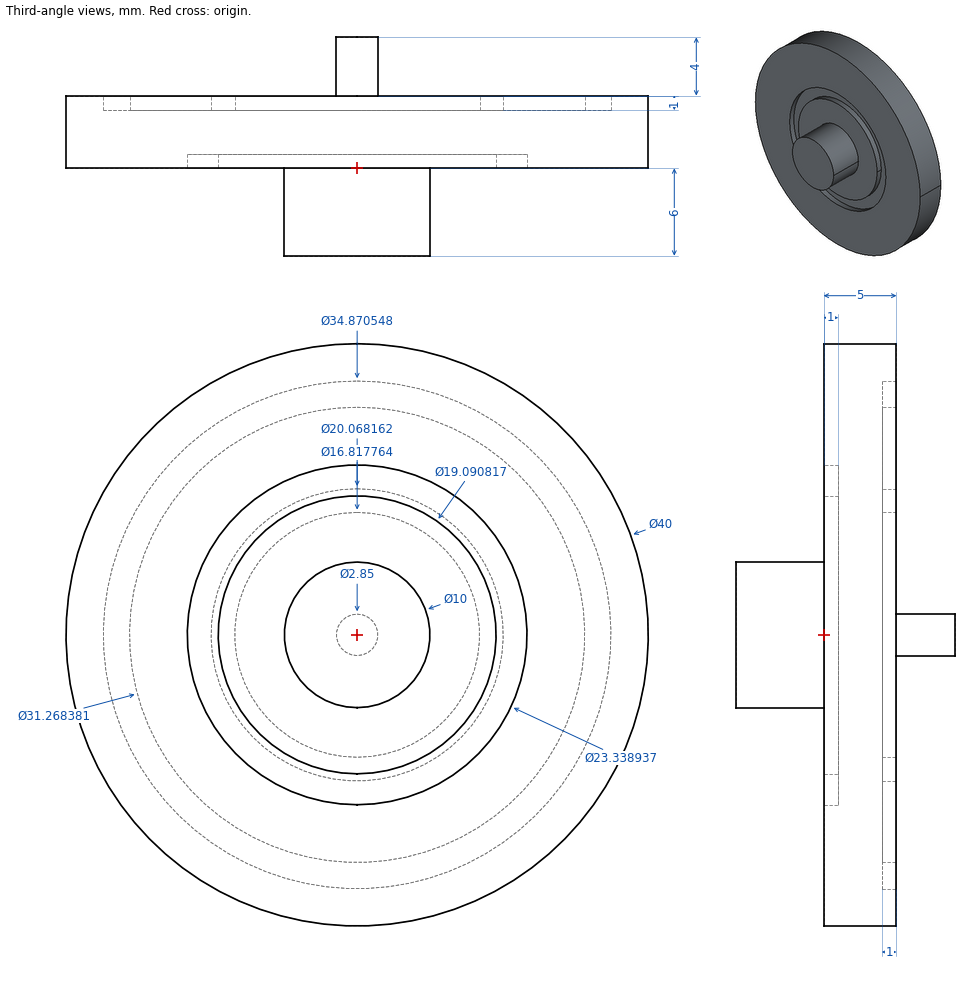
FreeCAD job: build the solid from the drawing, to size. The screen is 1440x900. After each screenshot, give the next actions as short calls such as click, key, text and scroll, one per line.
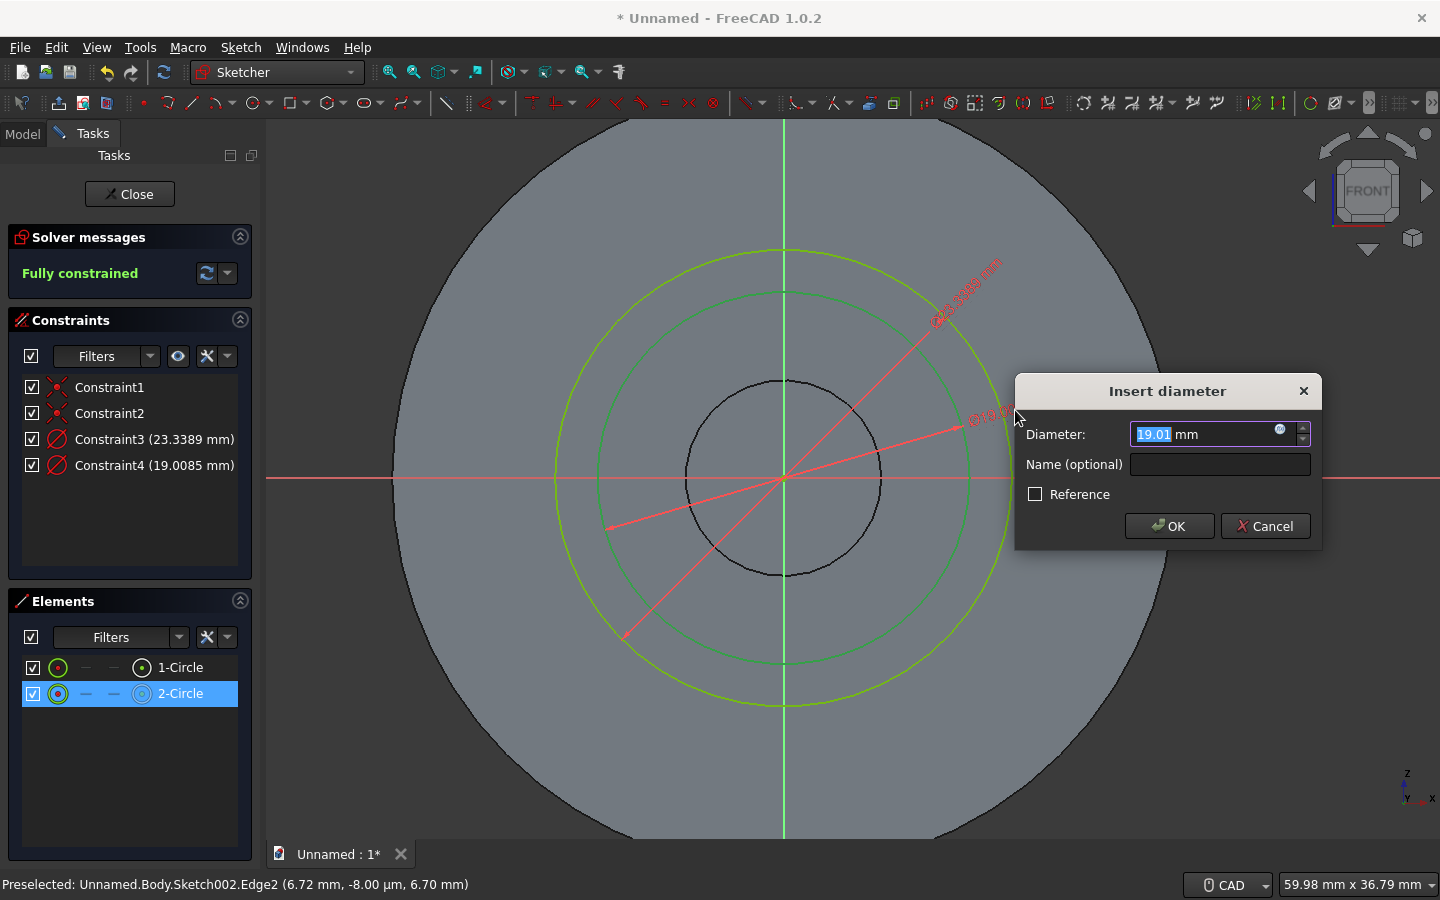
text(19.090817)
key(Return)
key(Escape)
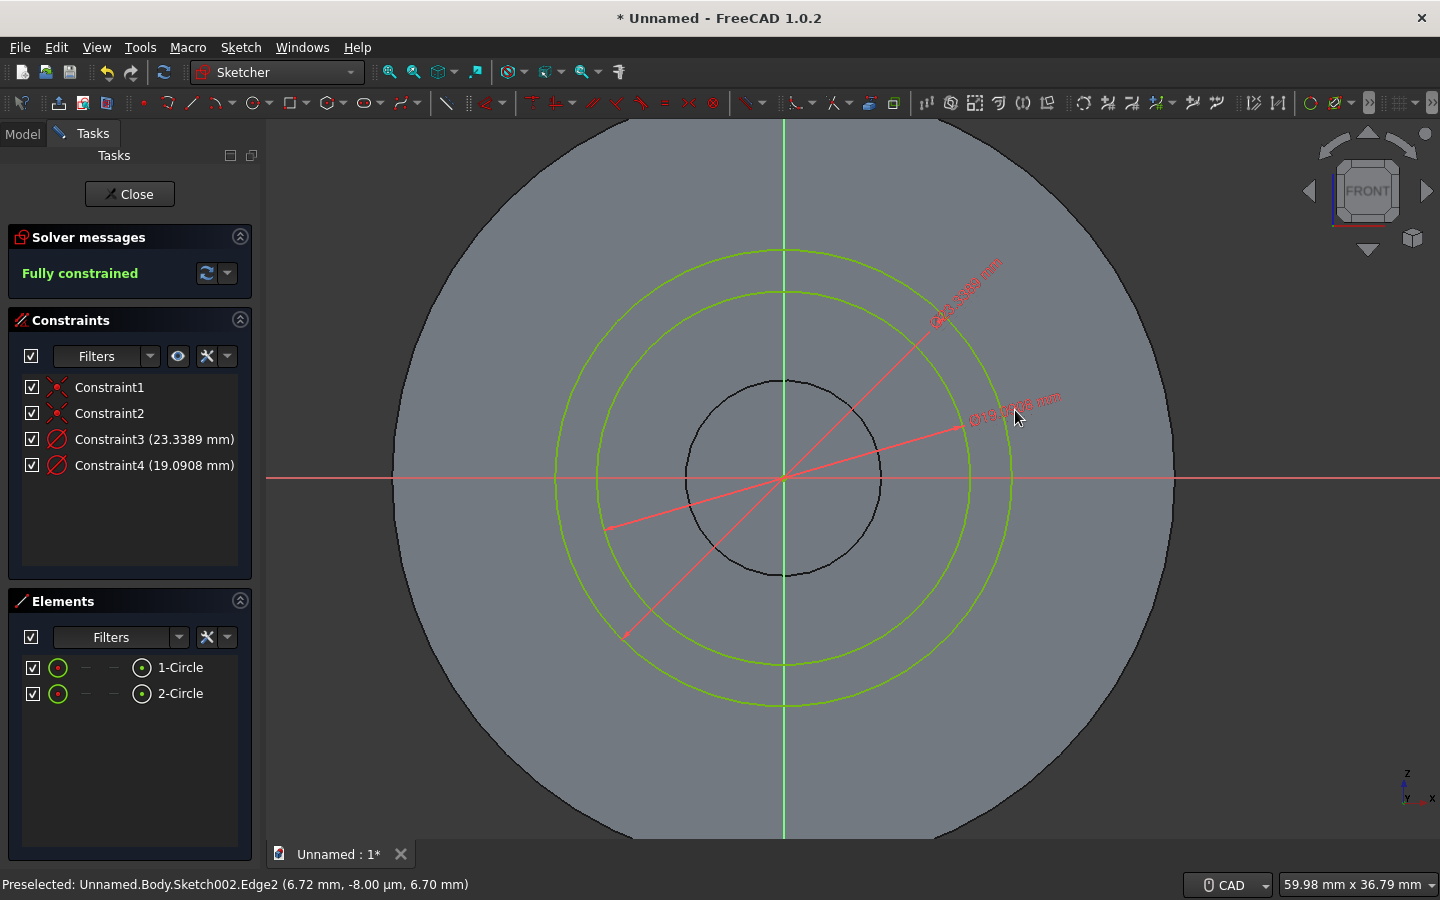
click(130, 194)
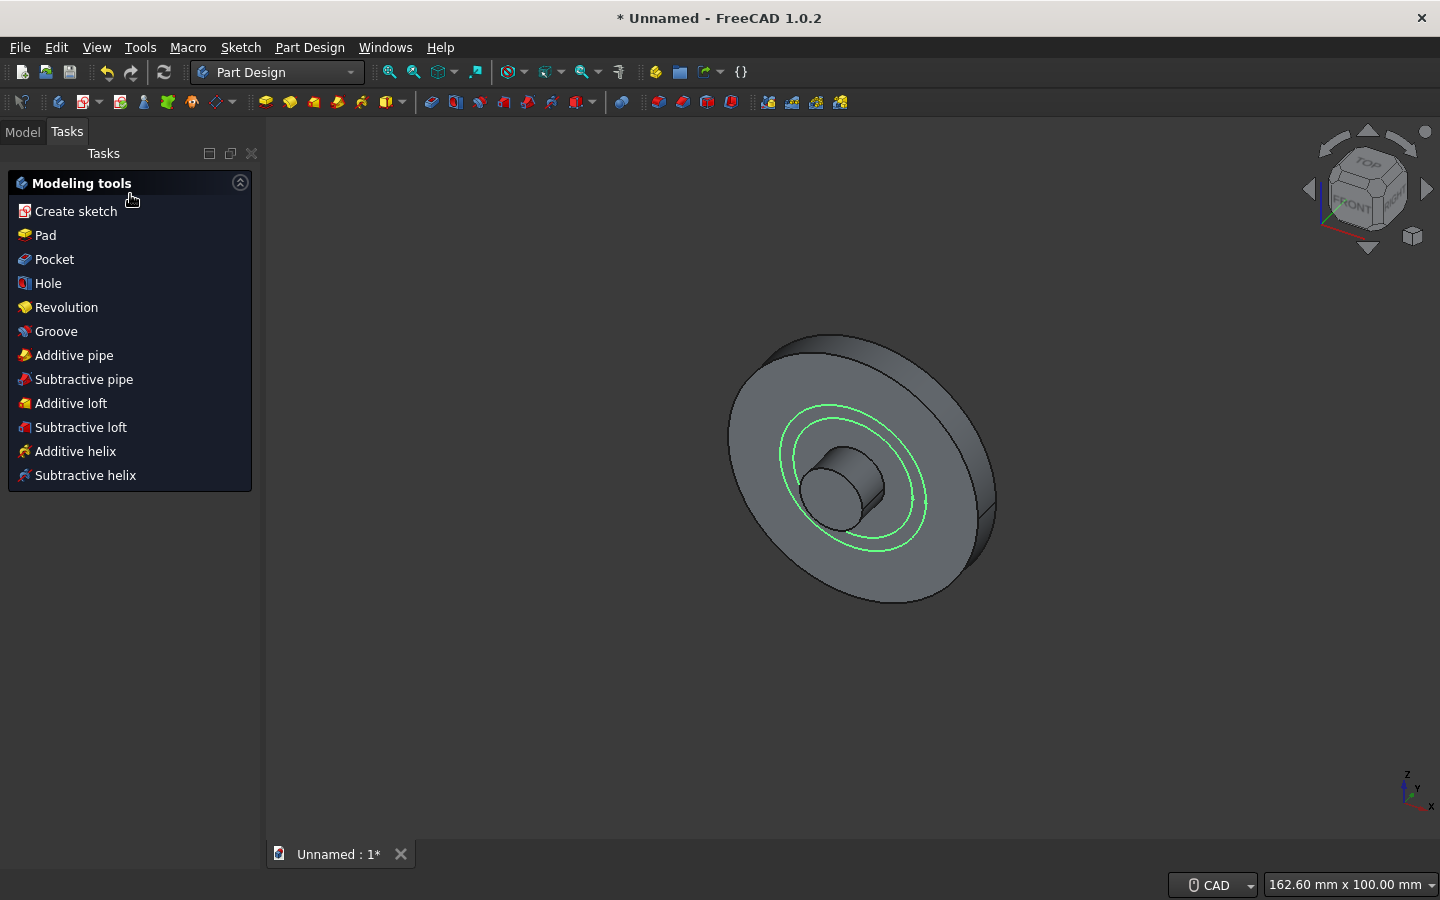
click(432, 102)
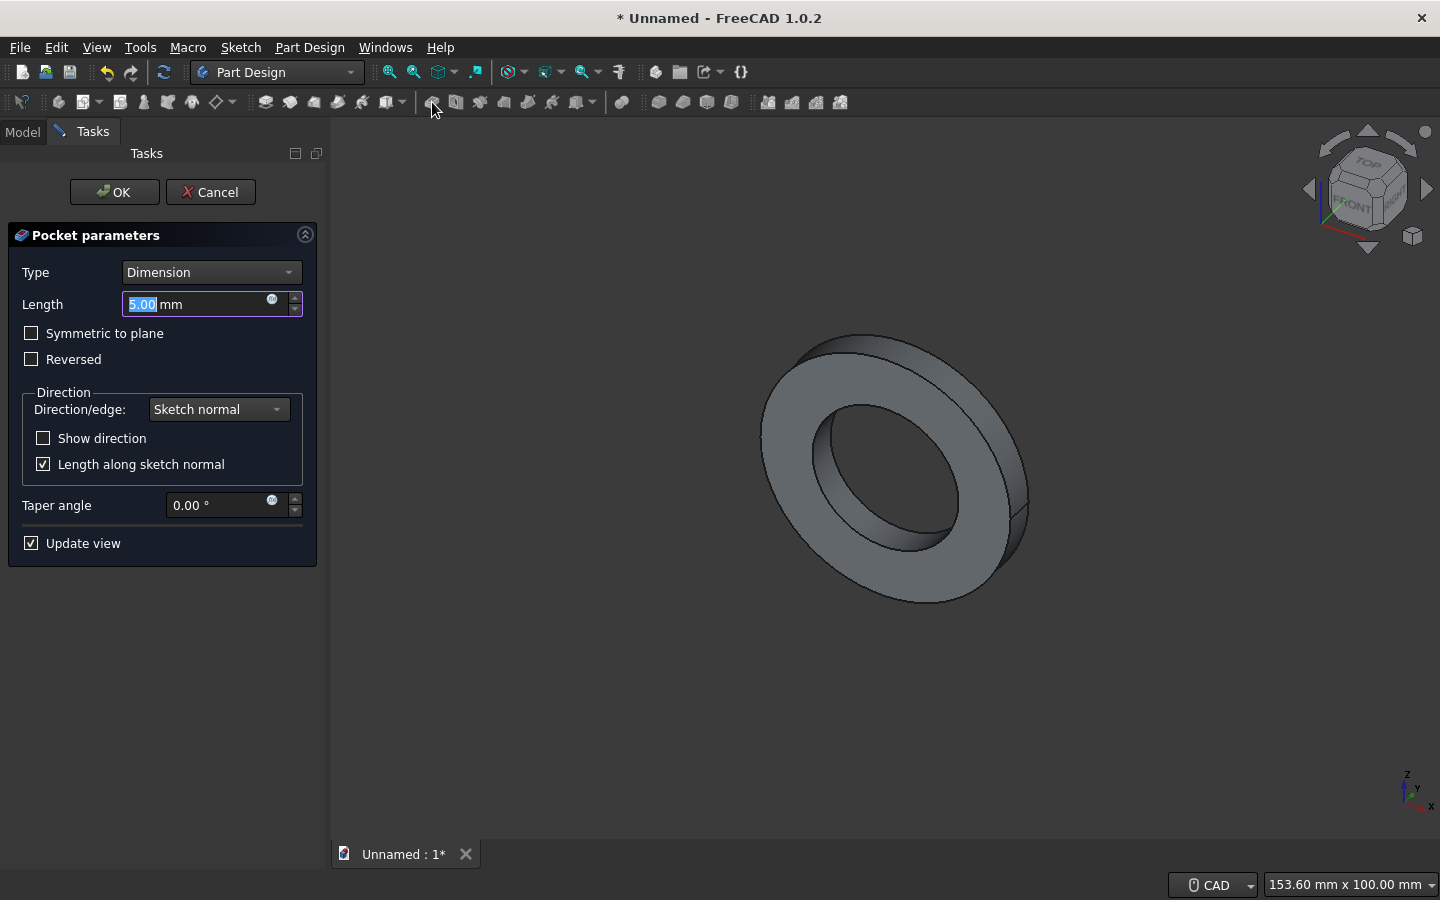
text(1)
key(Tab)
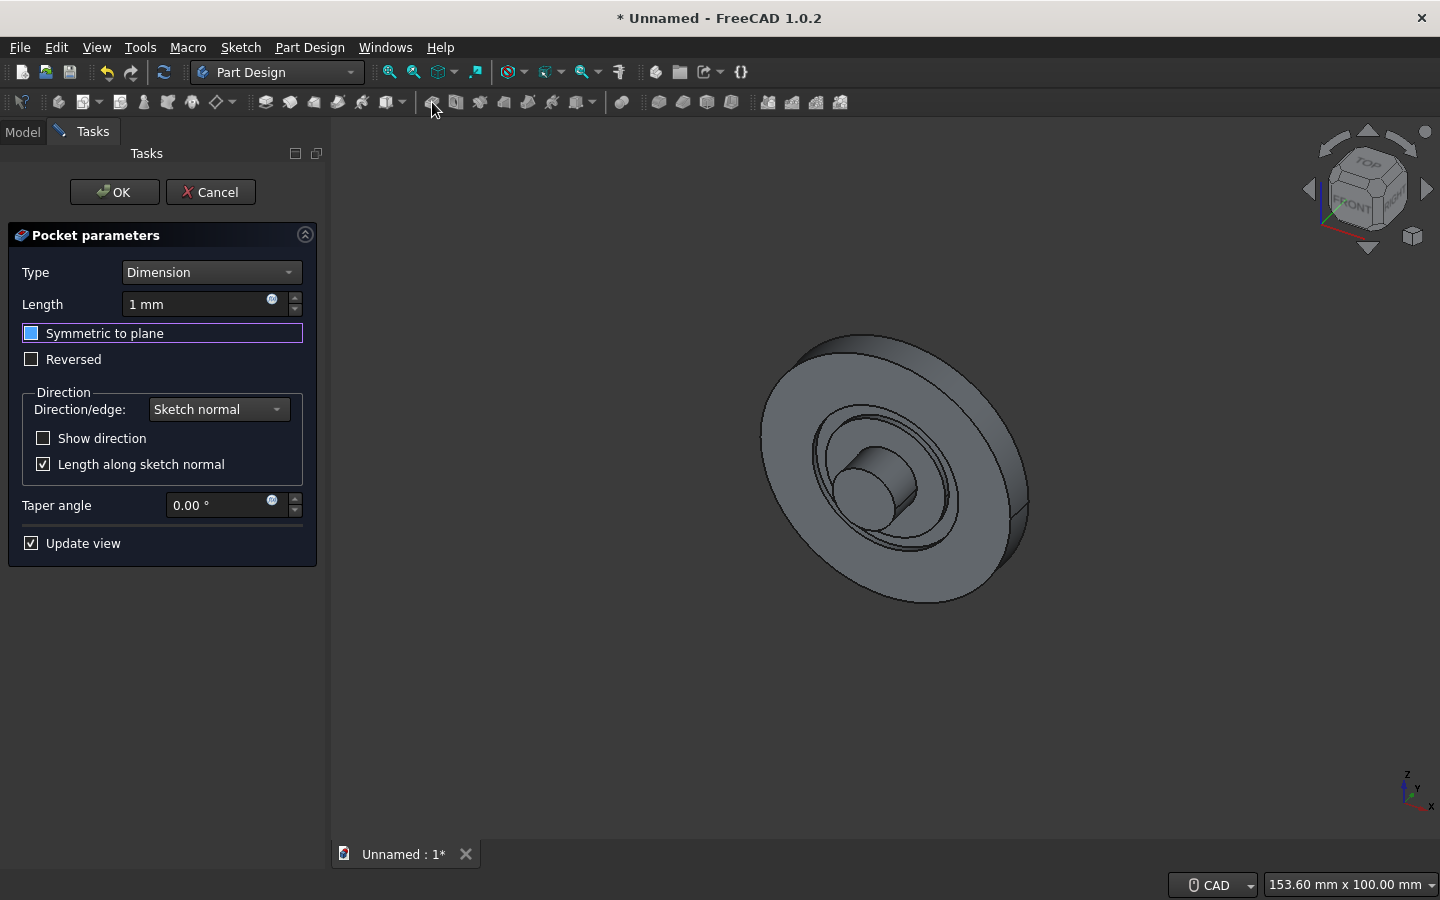
click(115, 192)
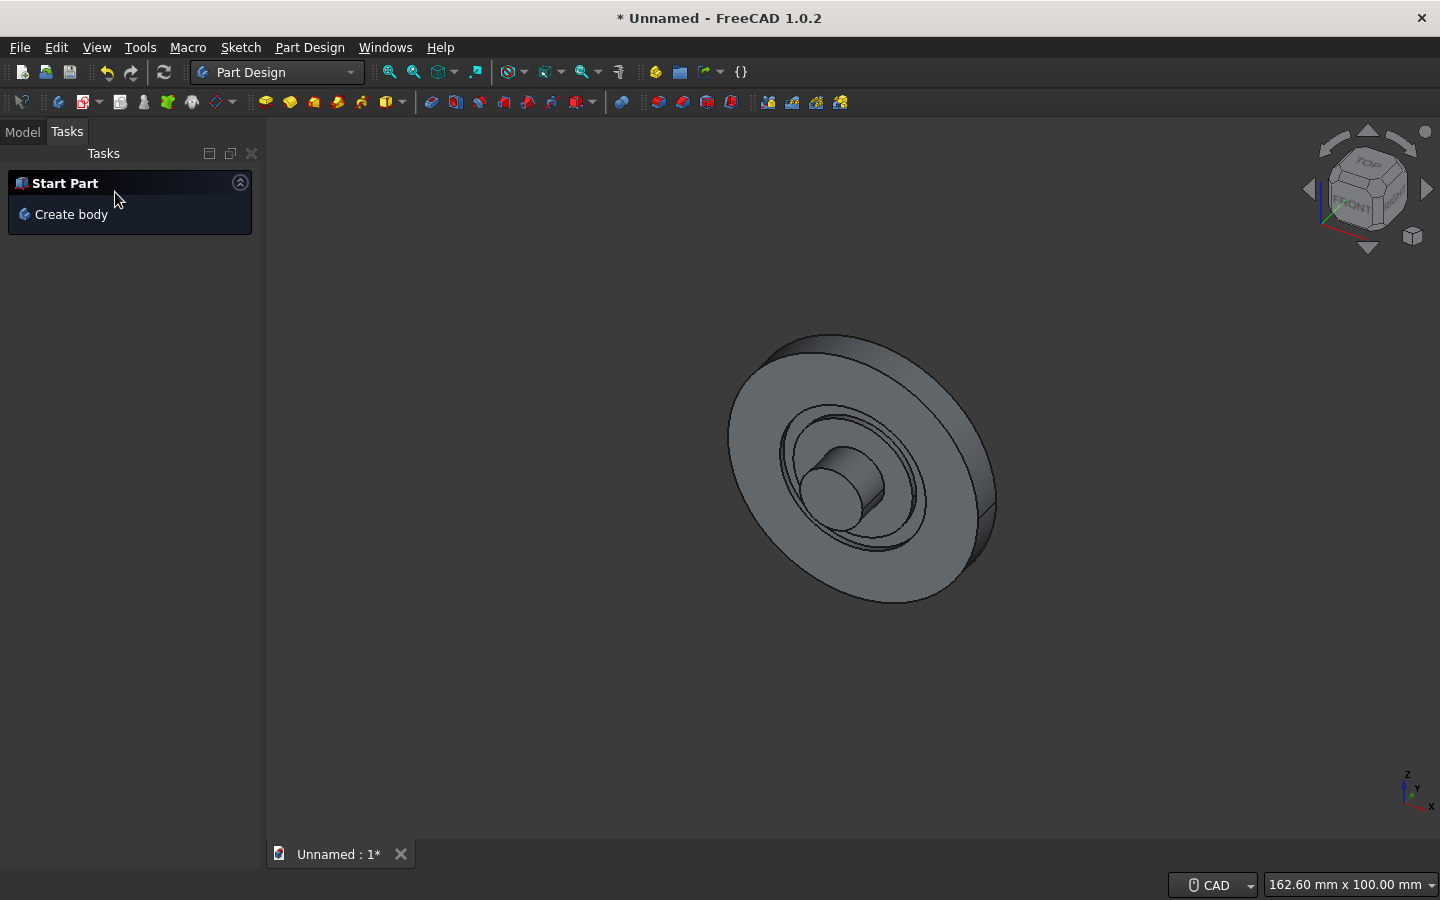
key(4)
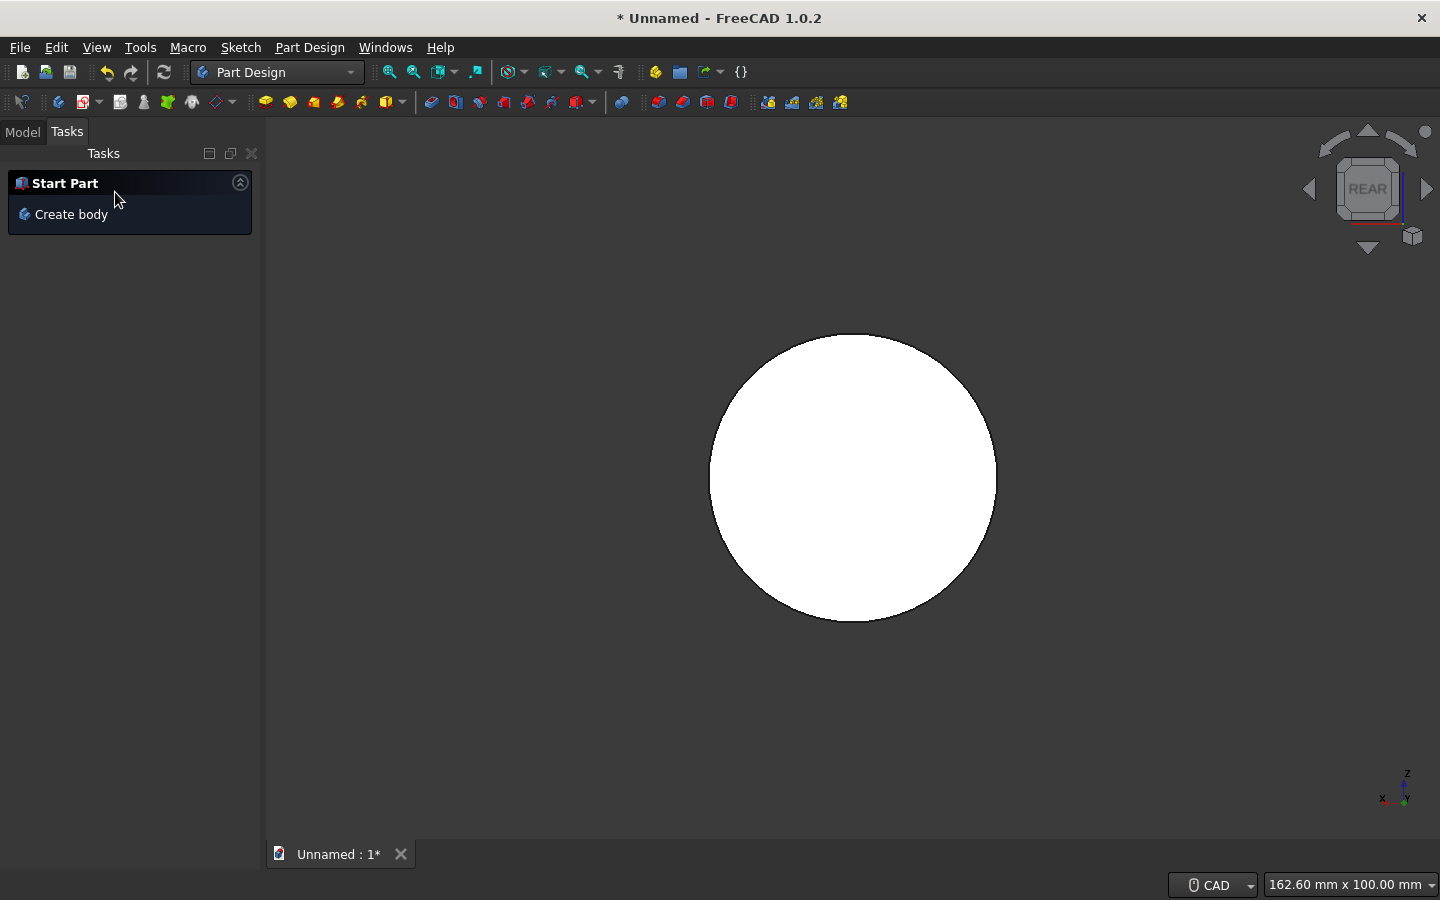
key(v)
key(f)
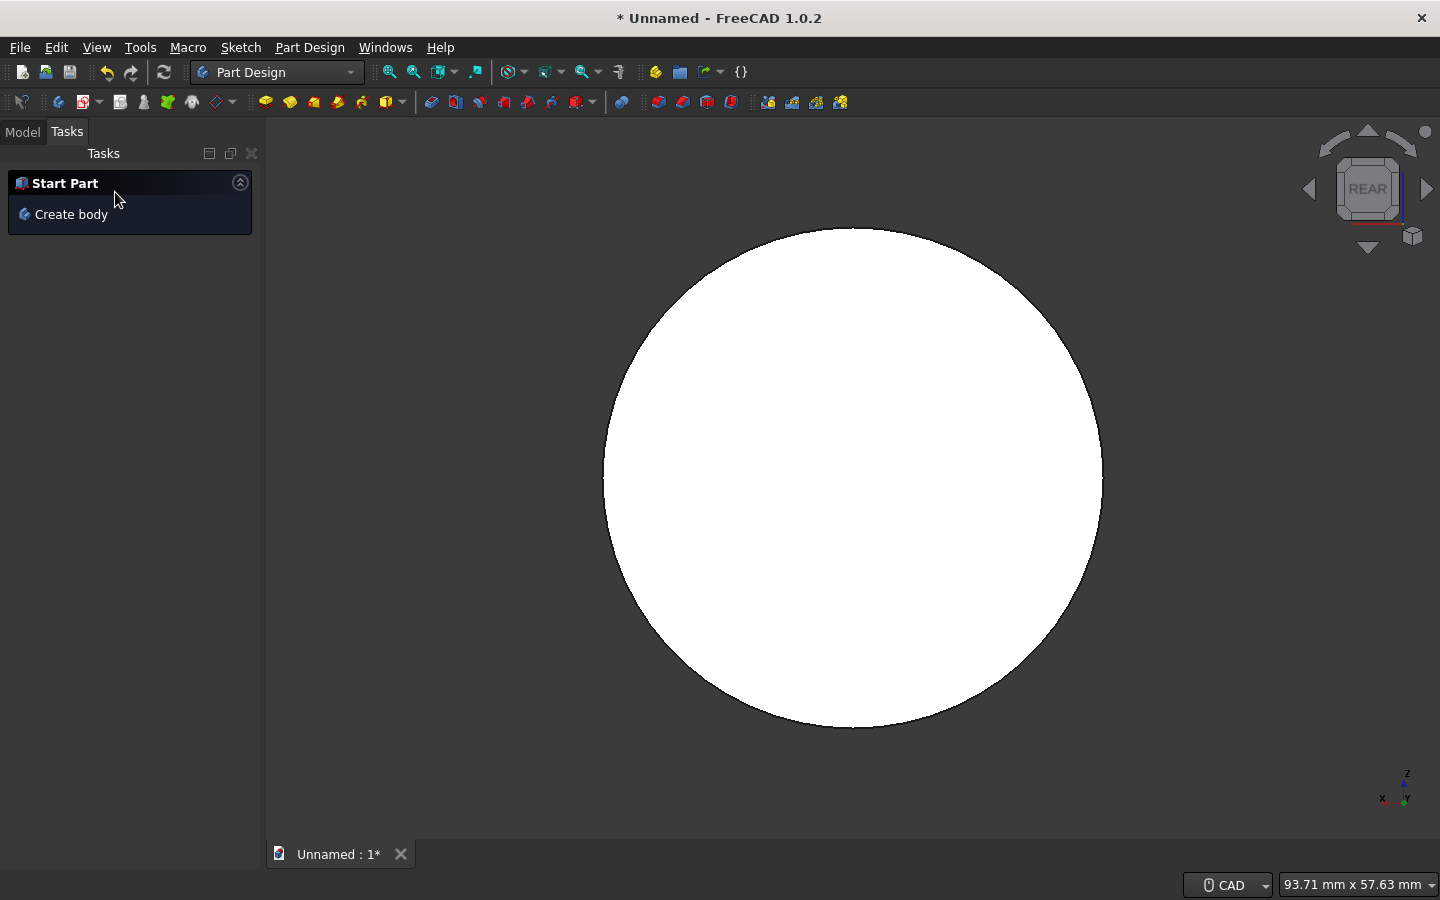
click(853, 477)